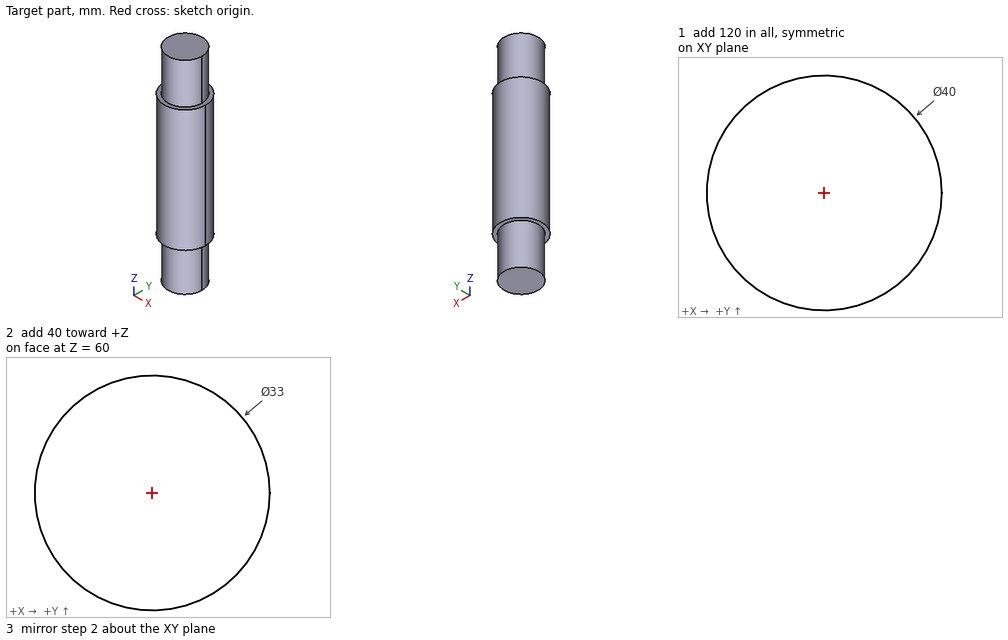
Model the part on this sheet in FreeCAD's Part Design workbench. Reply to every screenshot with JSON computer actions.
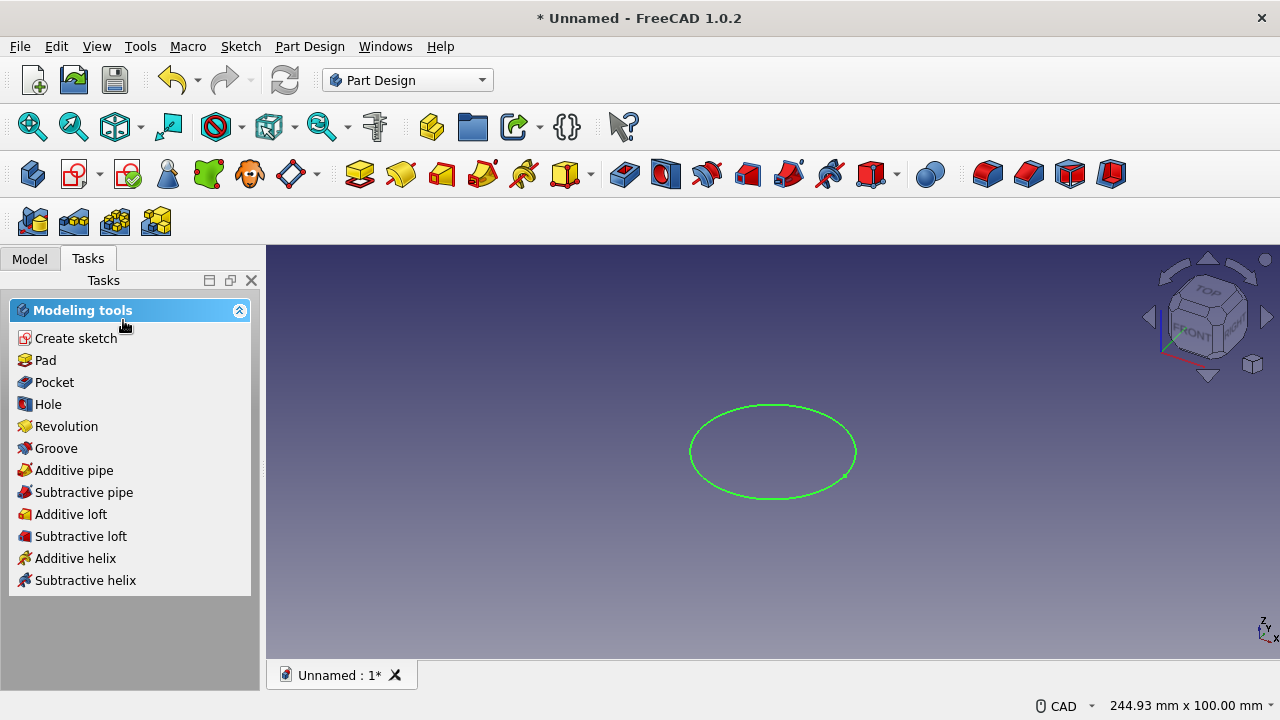
{"action": "left_click", "coordinate": [360, 174]}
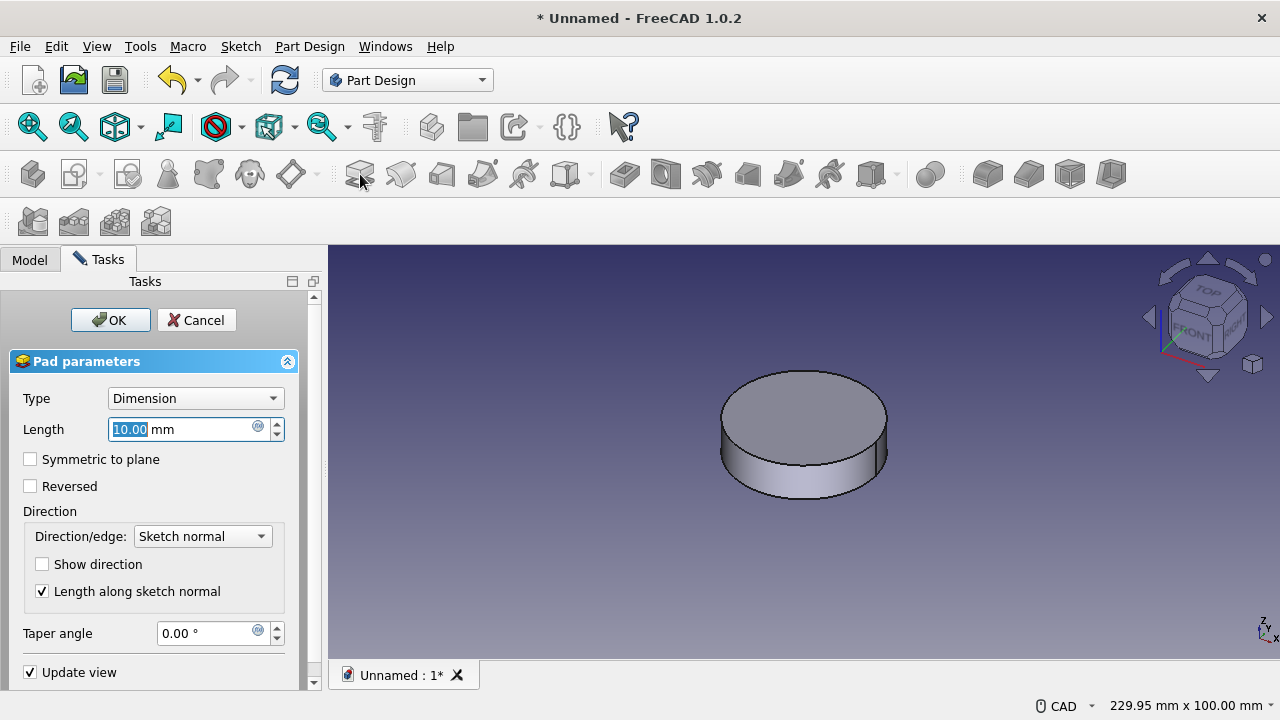
{"action": "type", "text": "120"}
{"action": "key", "text": "Tab"}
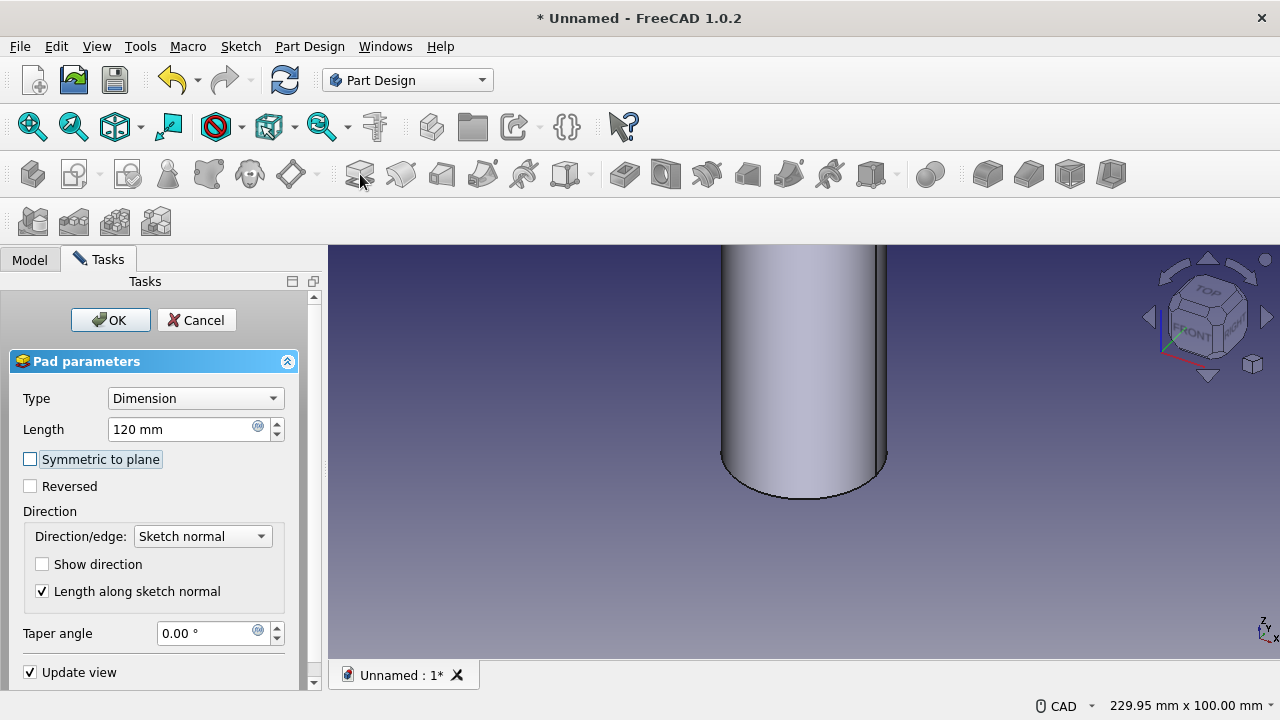
{"action": "left_click", "coordinate": [31, 459]}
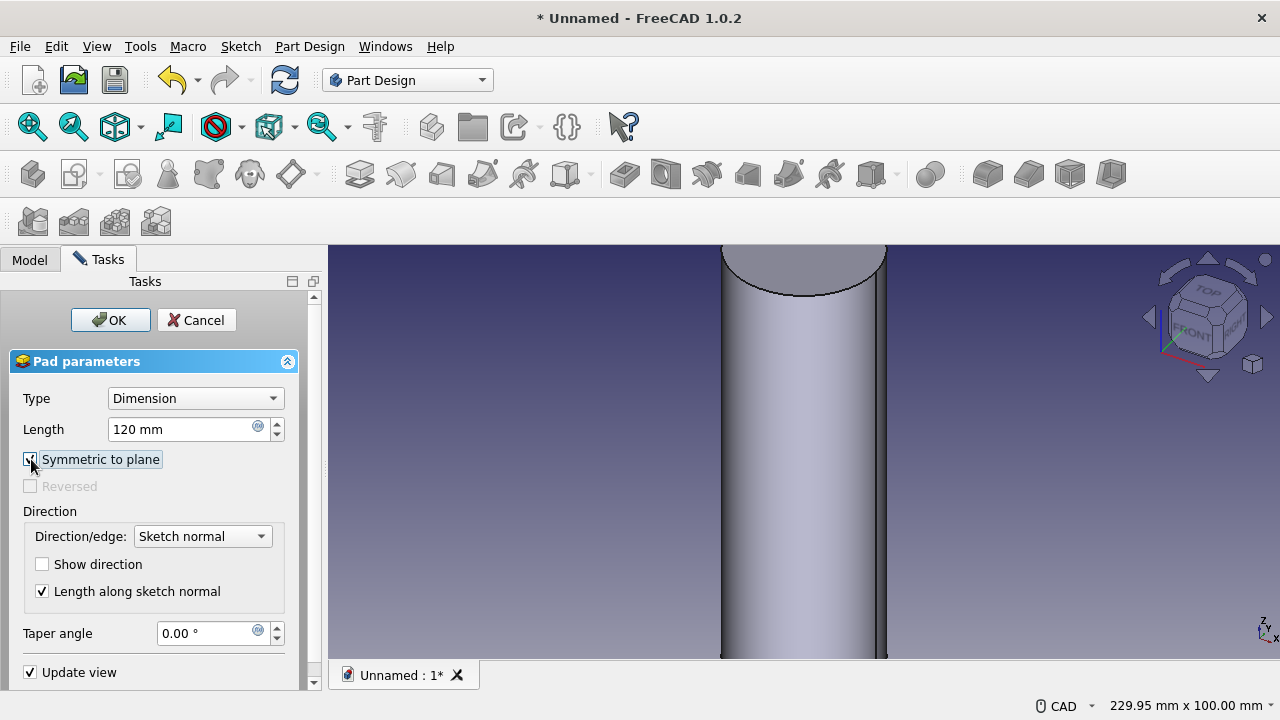
{"action": "left_click", "coordinate": [111, 320]}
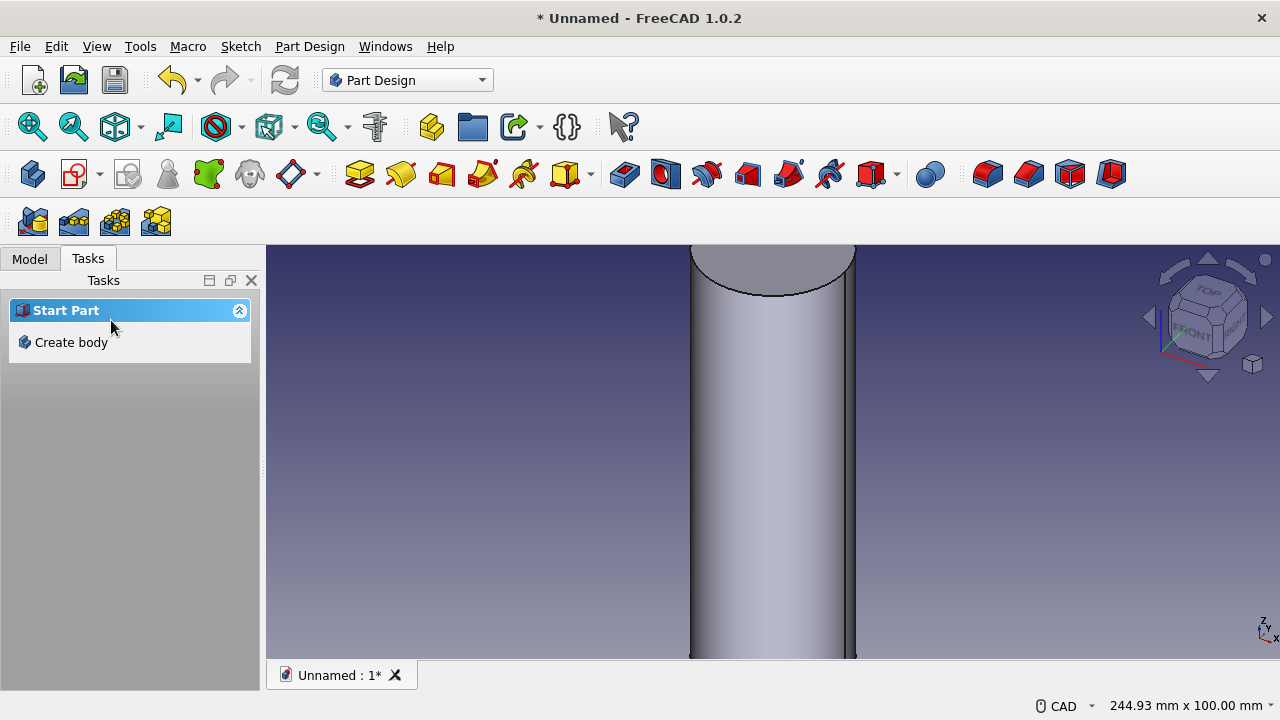
{"action": "left_click", "coordinate": [33, 128]}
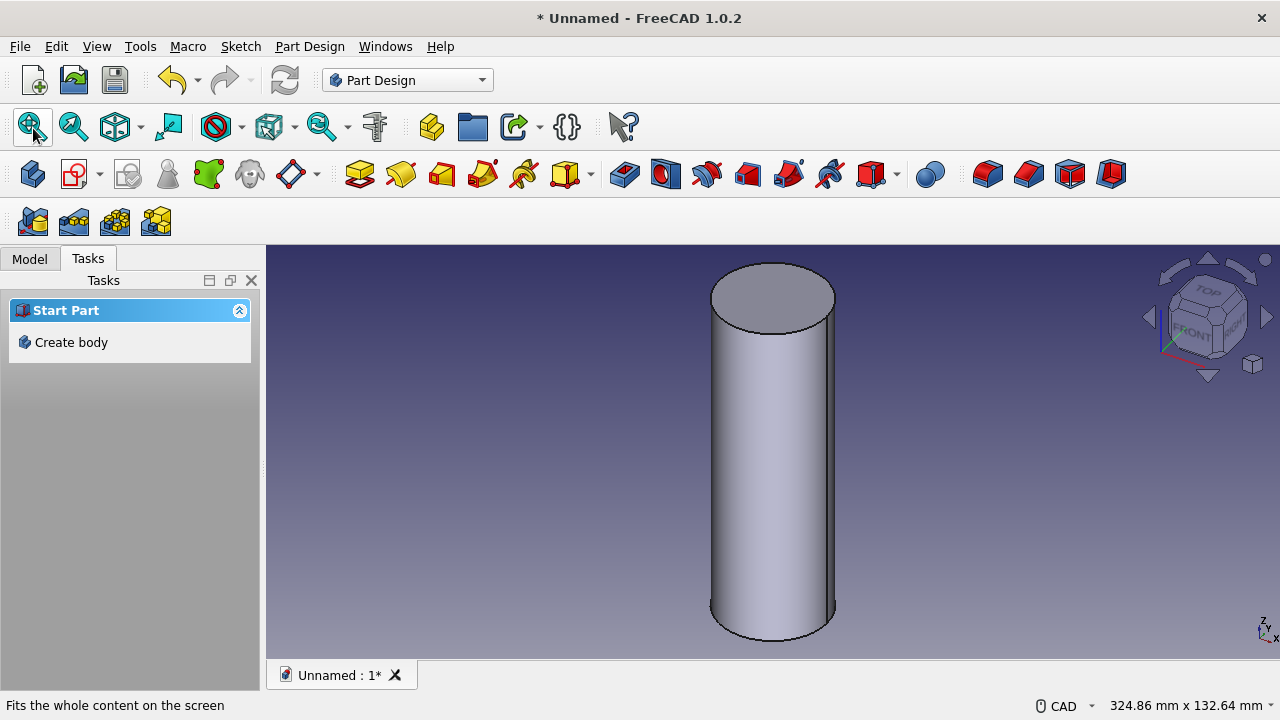
{"action": "left_click", "coordinate": [773, 298]}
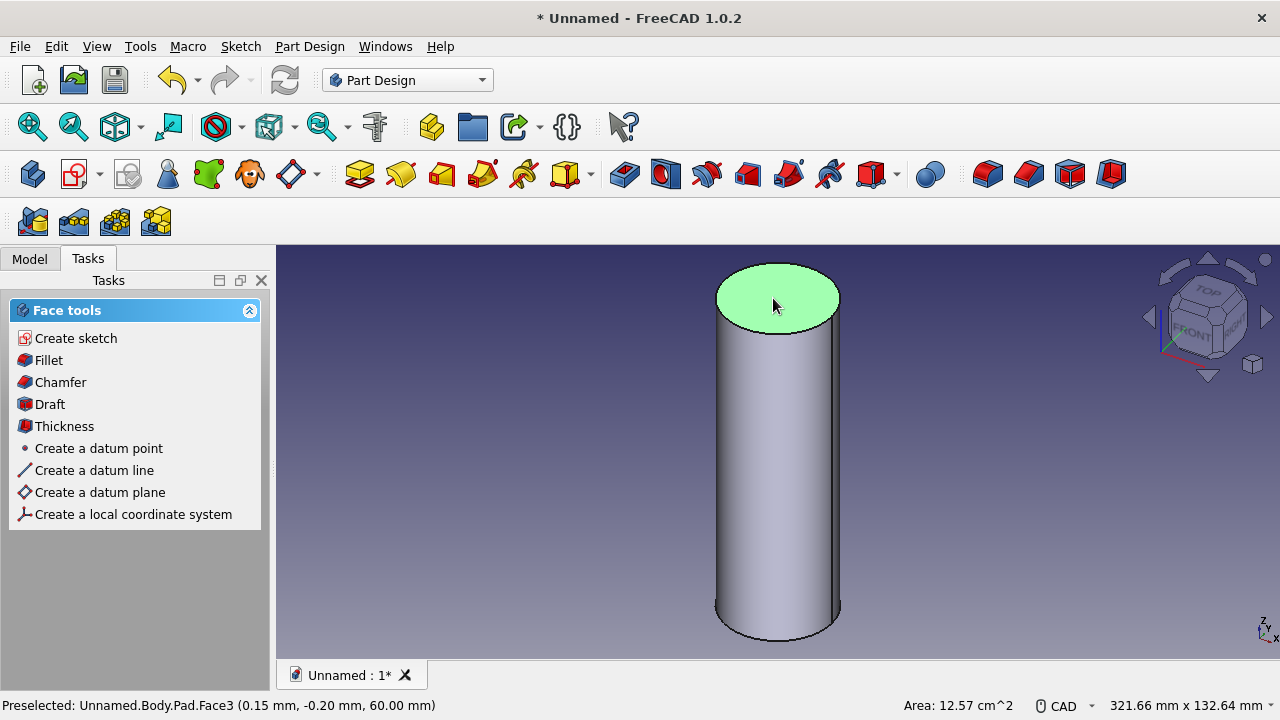
{"action": "left_click", "coordinate": [74, 174]}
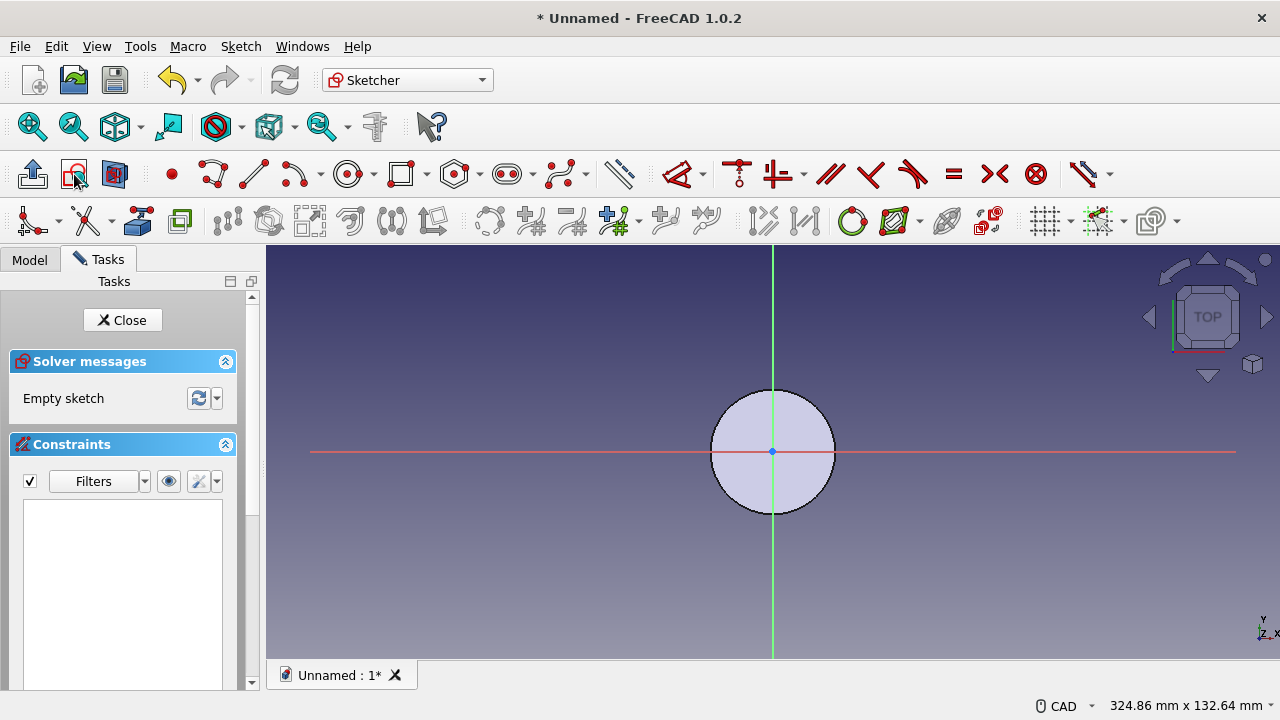
{"action": "scroll", "coordinate": [829, 452], "scroll_direction": "up", "scroll_amount": 4}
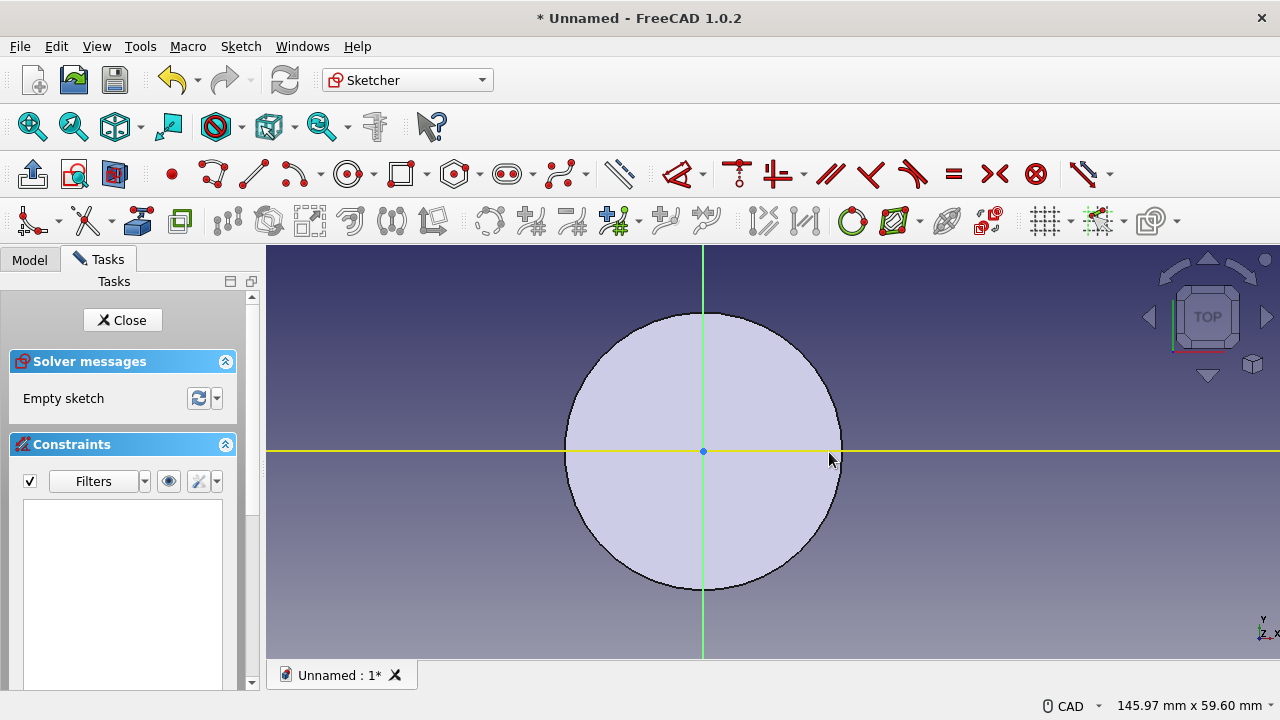
{"action": "left_click", "coordinate": [348, 174]}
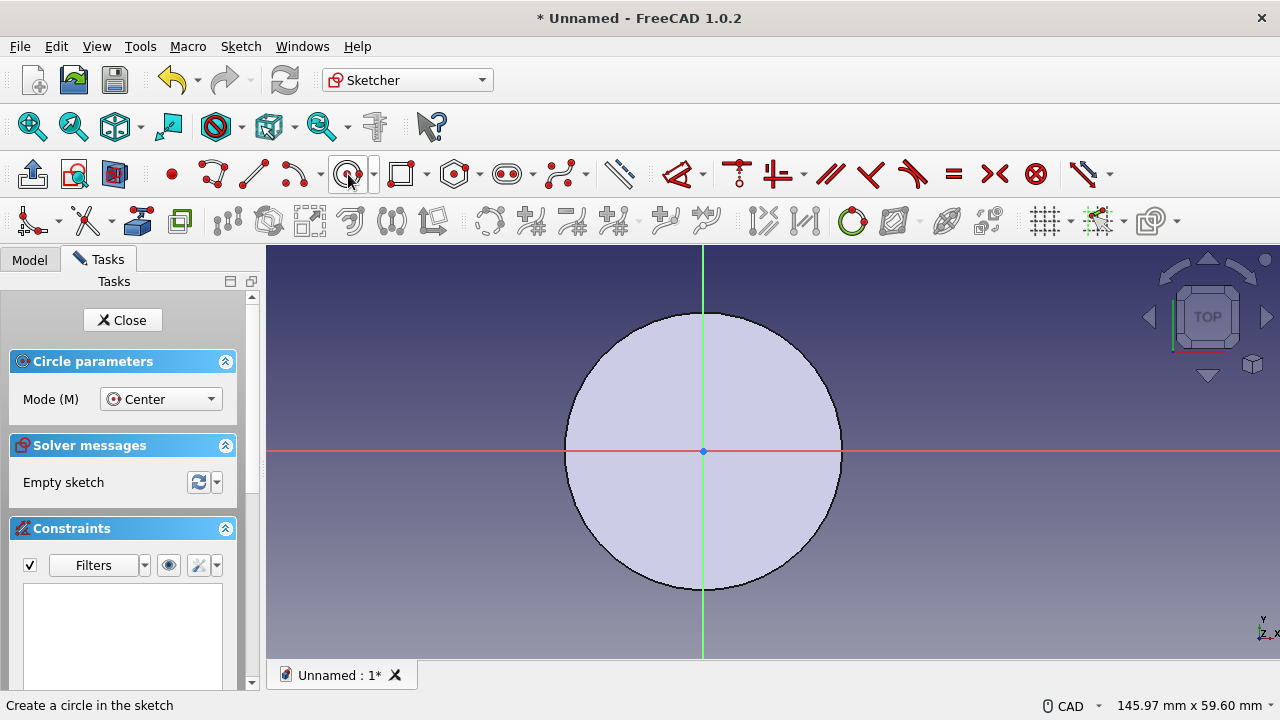
{"action": "left_click", "coordinate": [703, 451]}
{"action": "left_click", "coordinate": [785, 370]}
{"action": "key", "text": "Escape"}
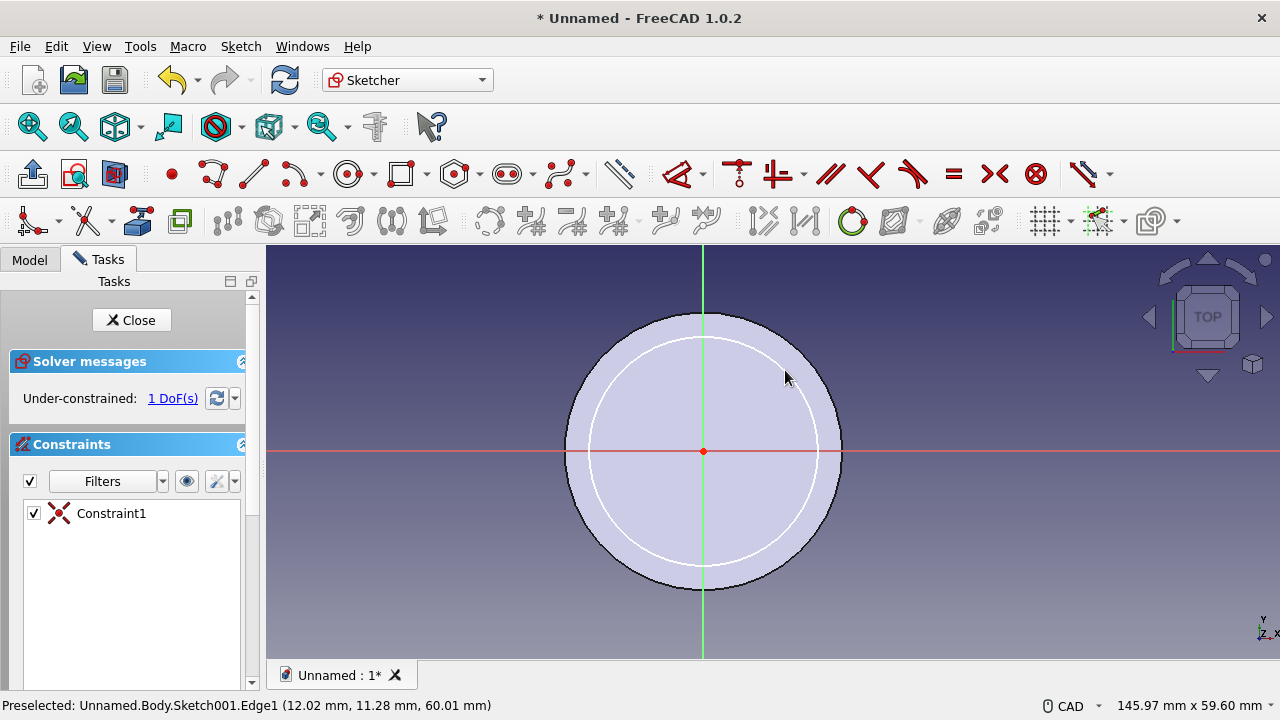
{"action": "left_click", "coordinate": [784, 370]}